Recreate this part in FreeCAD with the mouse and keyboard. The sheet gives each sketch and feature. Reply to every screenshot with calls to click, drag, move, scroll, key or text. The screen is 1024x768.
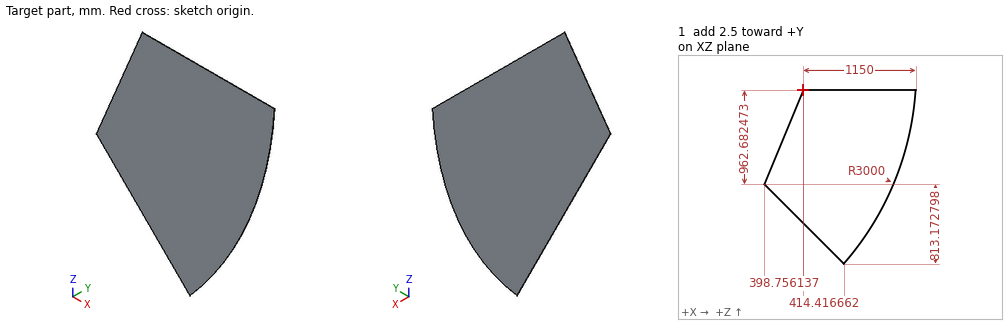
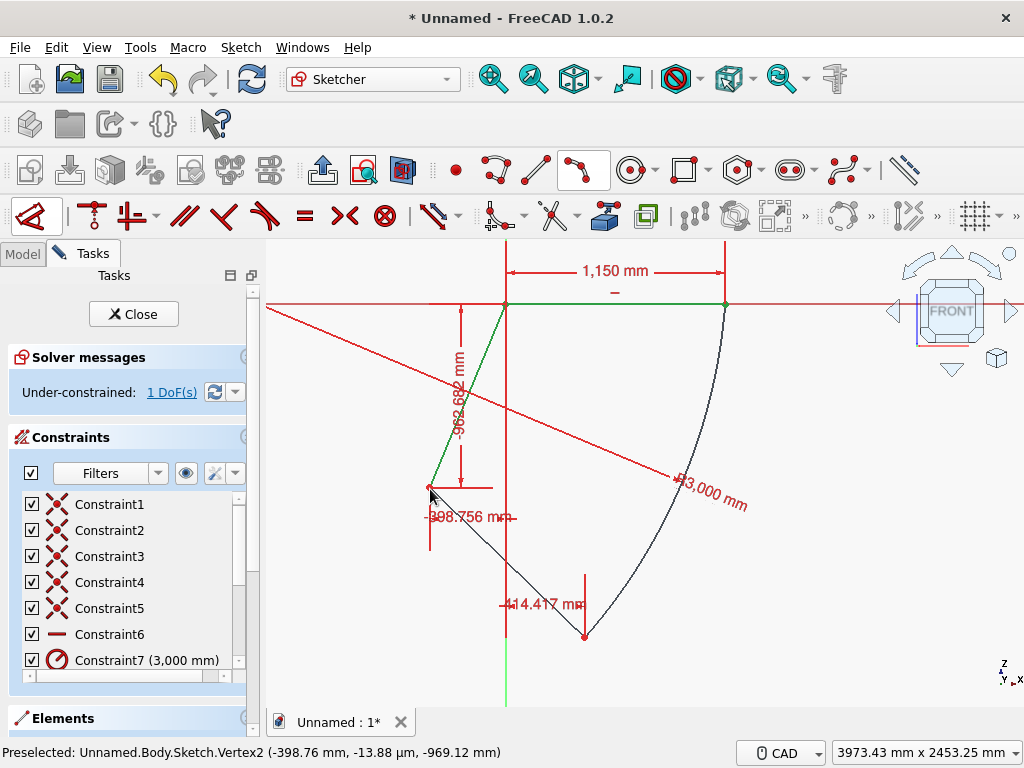
click(538, 593)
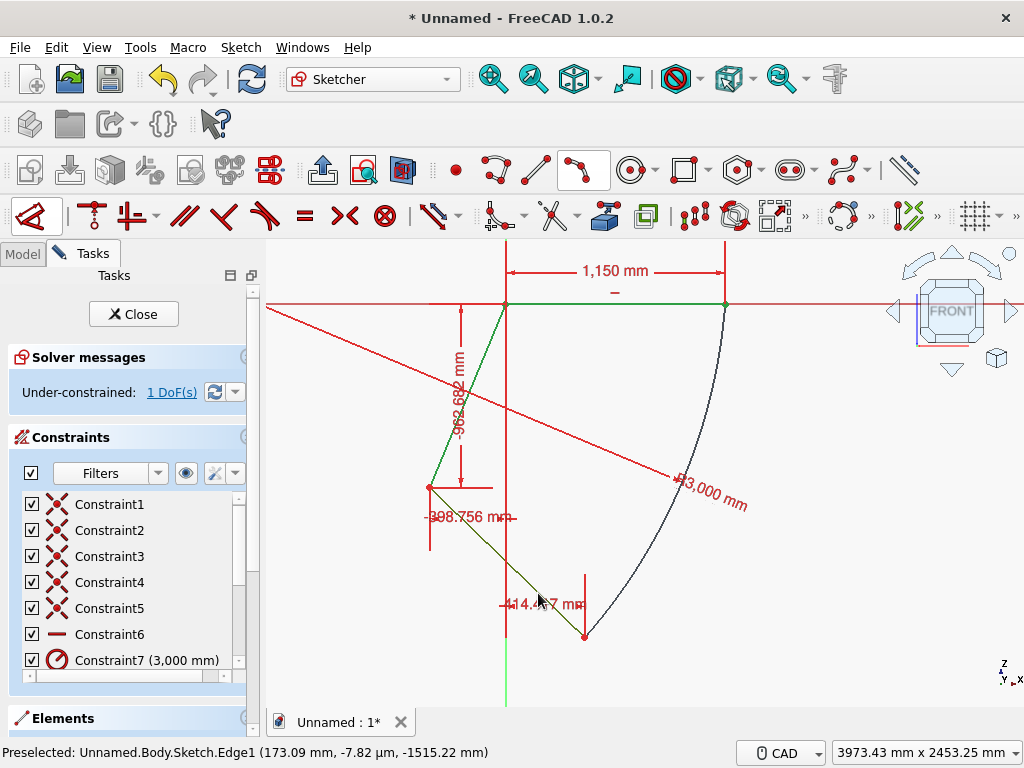
key(i)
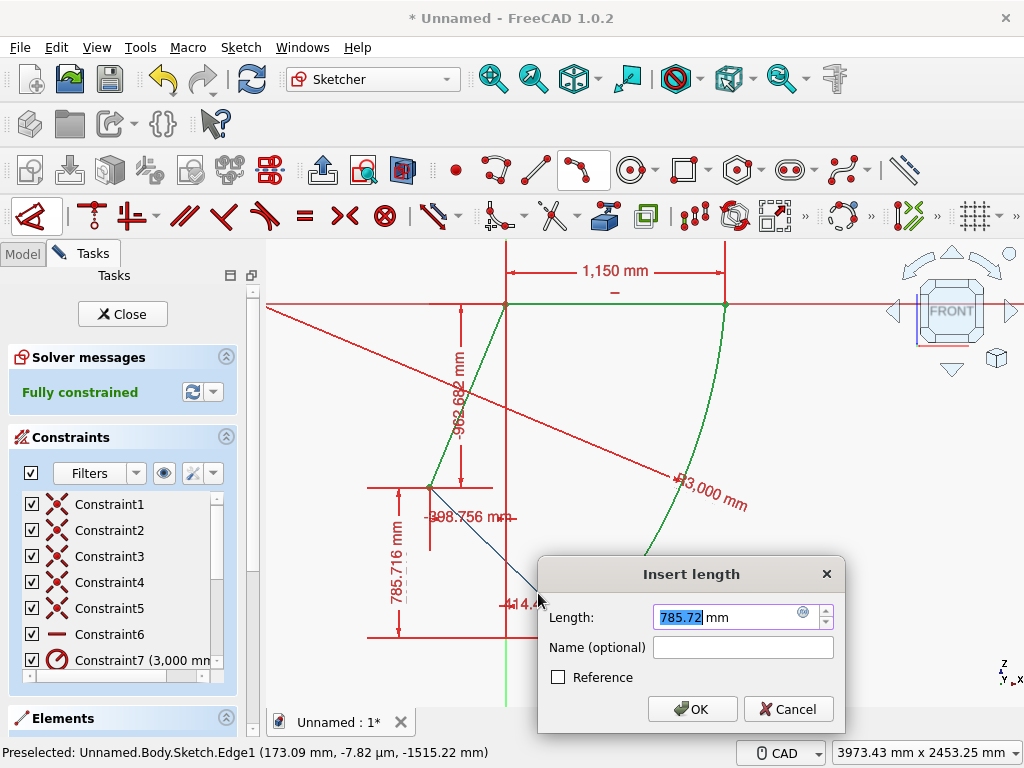
text(813.172798)
key(Return)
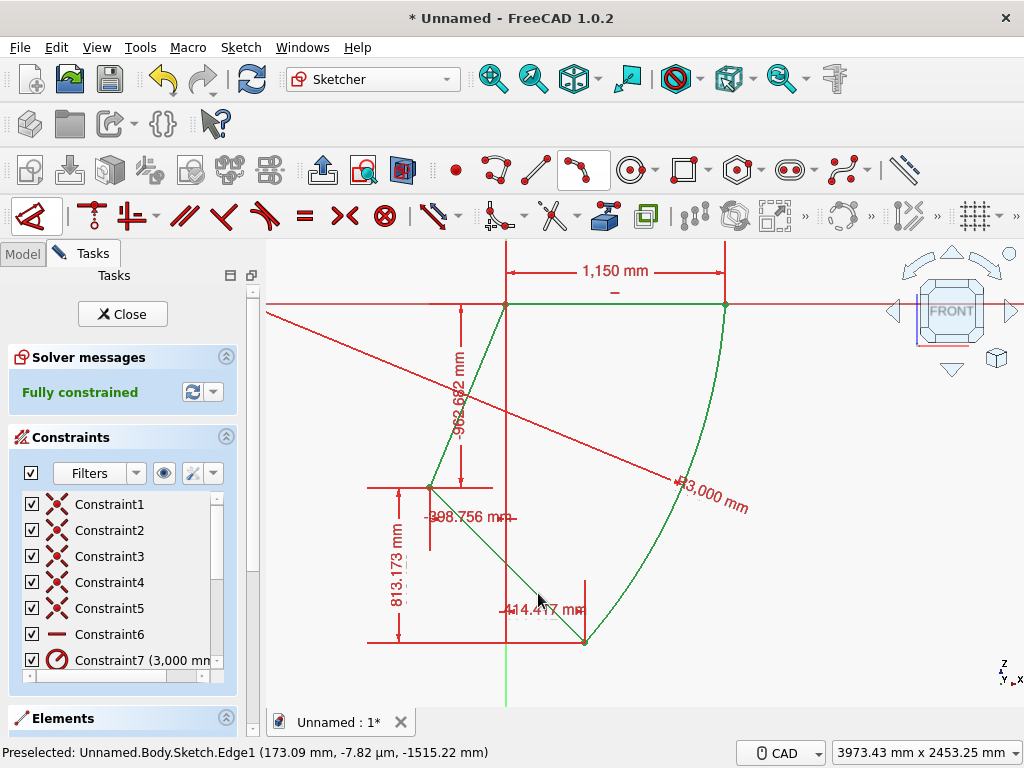
click(123, 314)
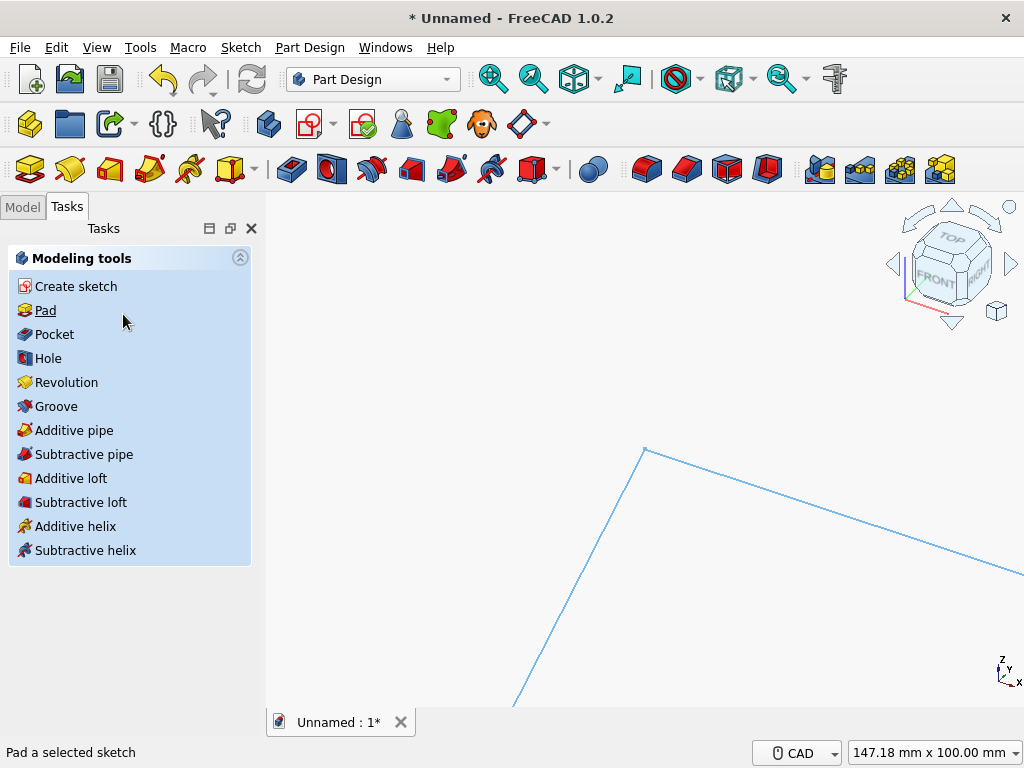
click(30, 170)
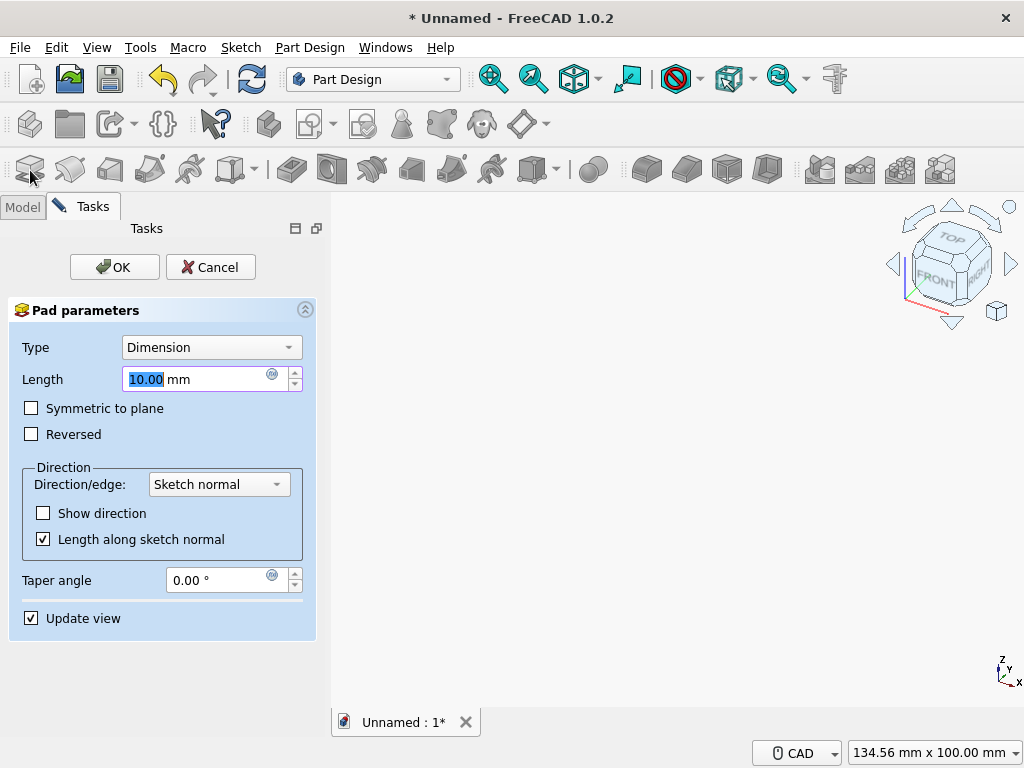
text(2.5)
key(Tab)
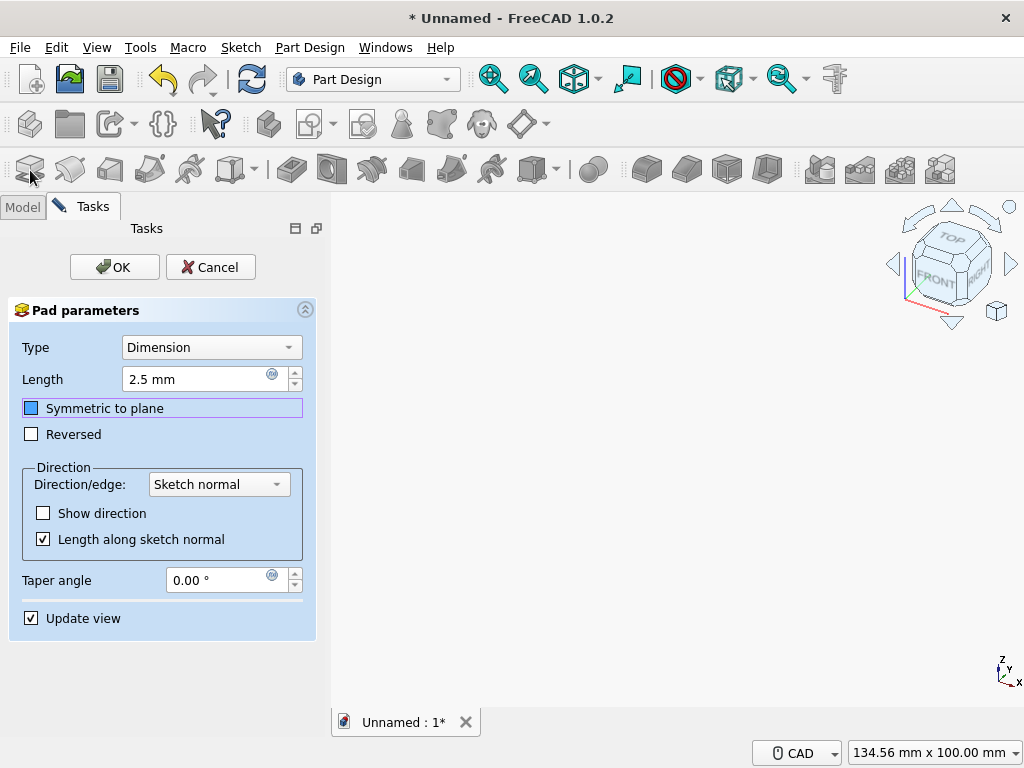
click(30, 434)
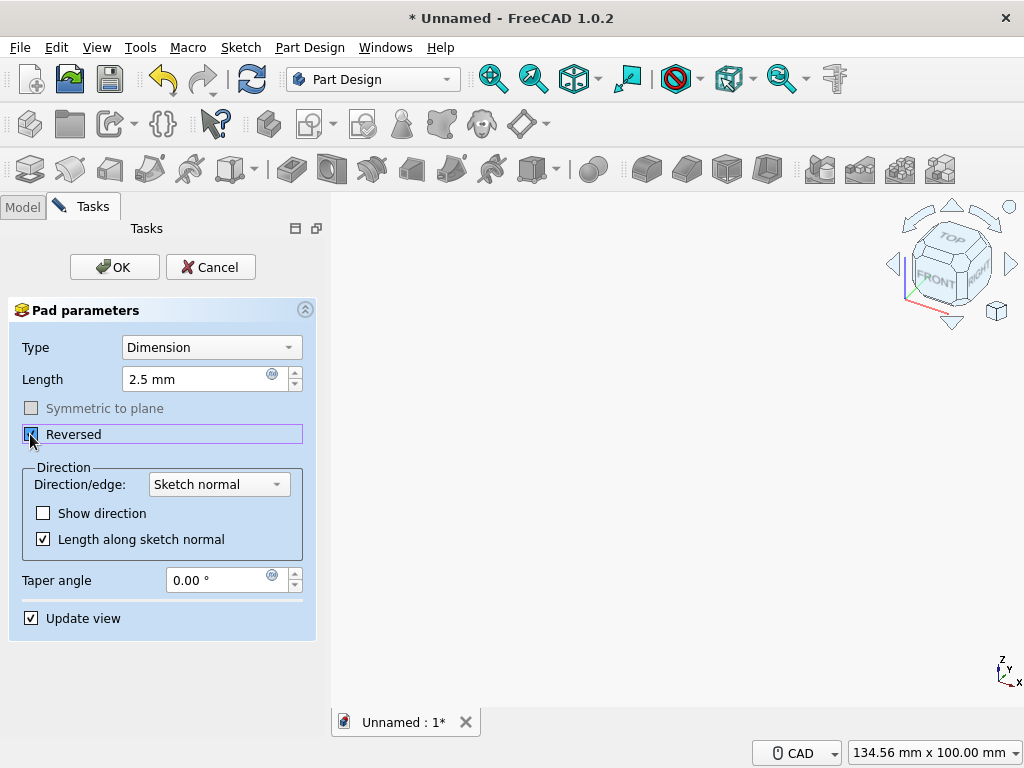
click(115, 267)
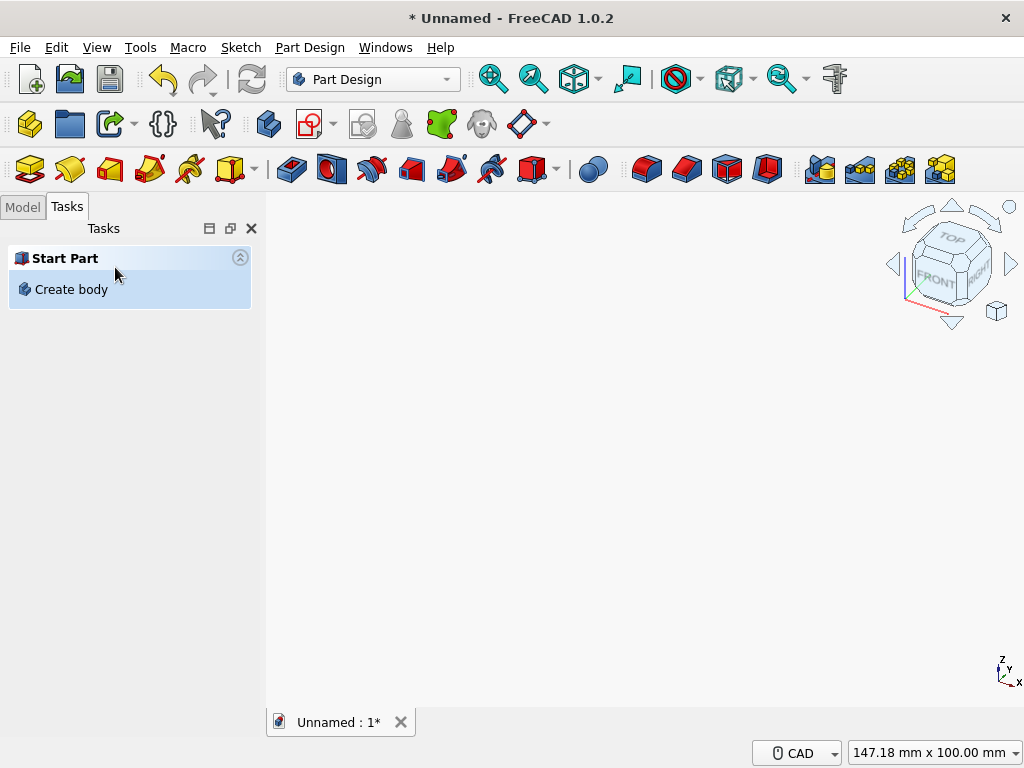
key(0)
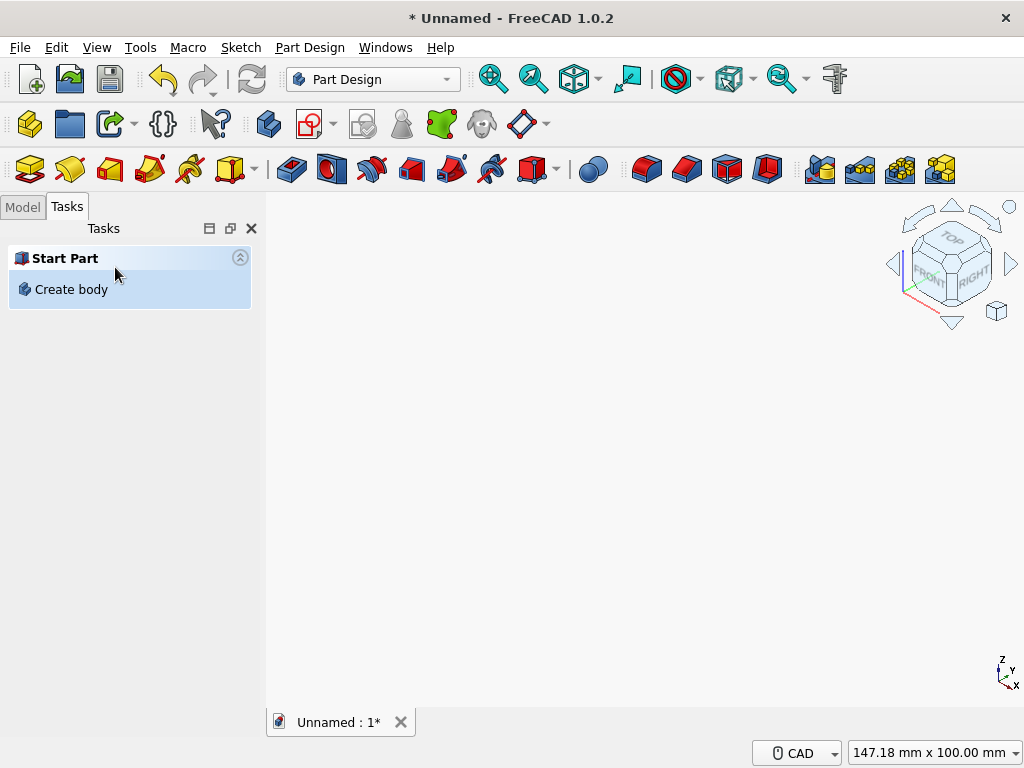
click(494, 80)